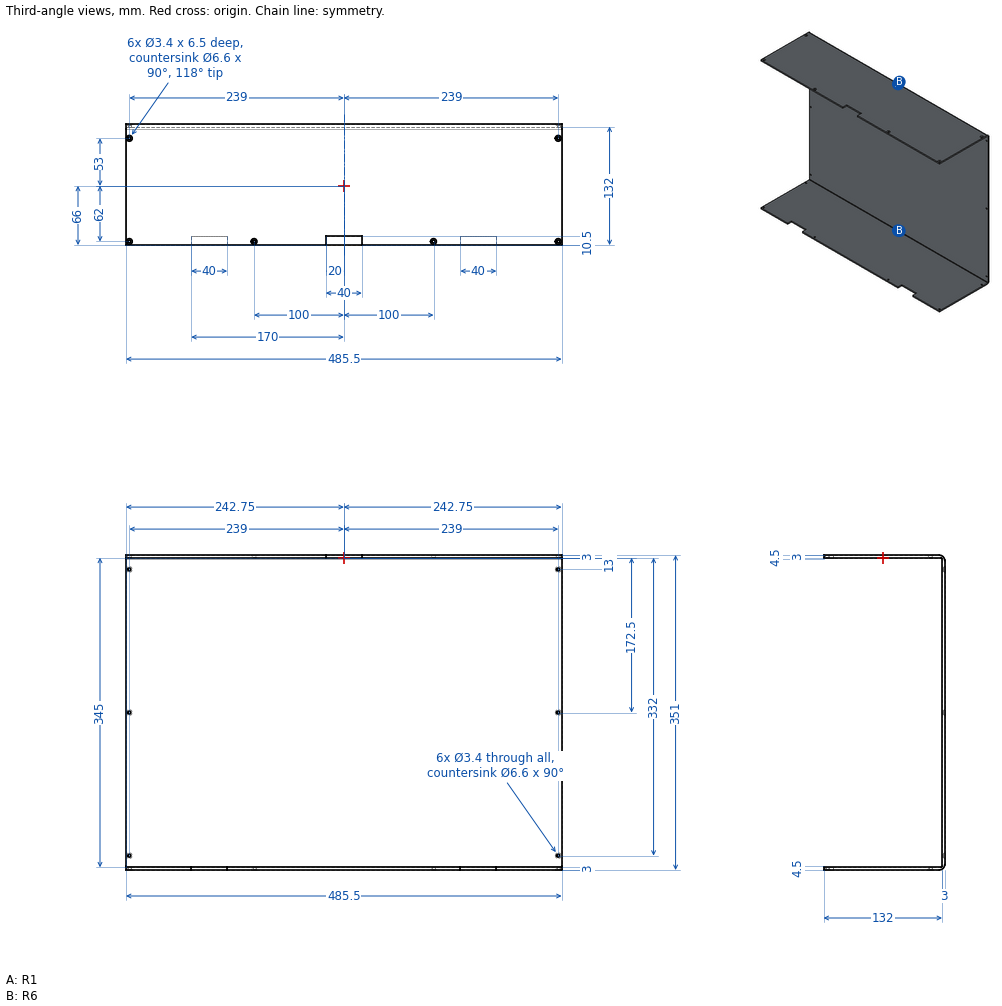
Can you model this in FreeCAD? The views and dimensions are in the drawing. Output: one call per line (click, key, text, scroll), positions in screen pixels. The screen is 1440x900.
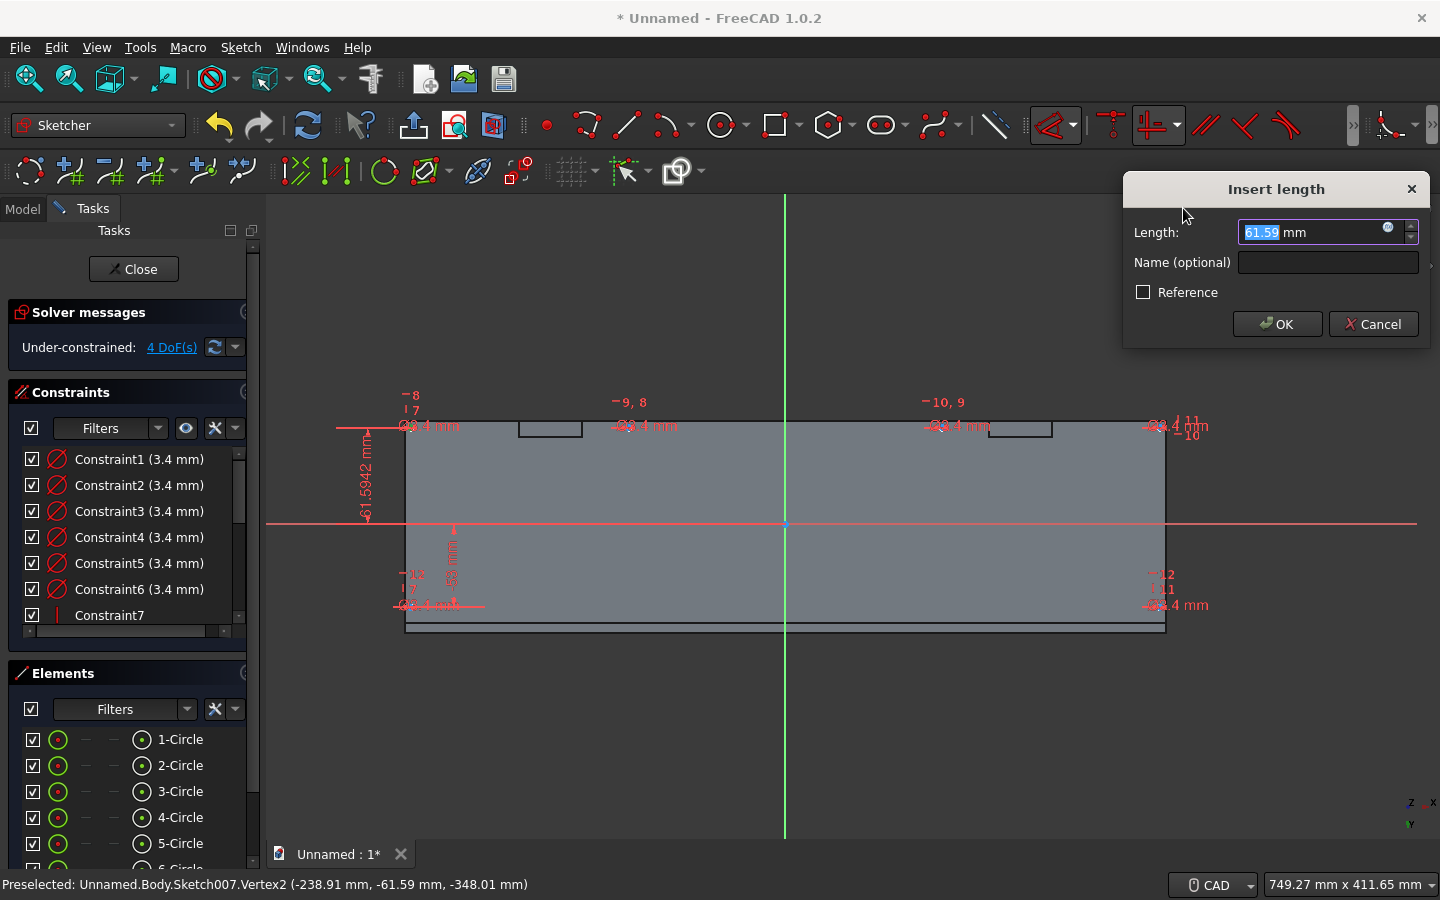
text(62)
key(Return)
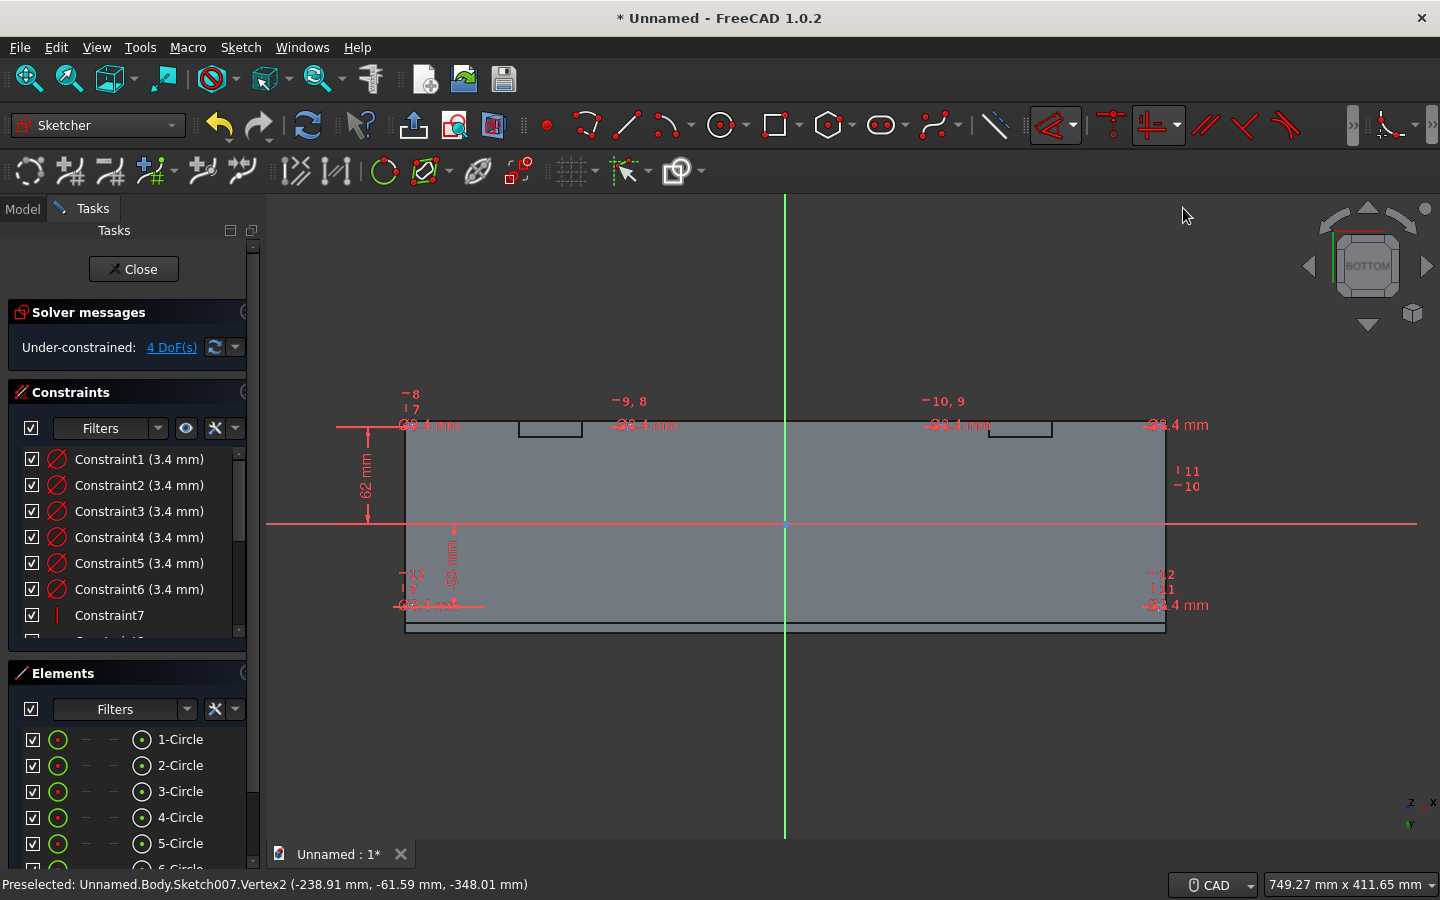
click(411, 607)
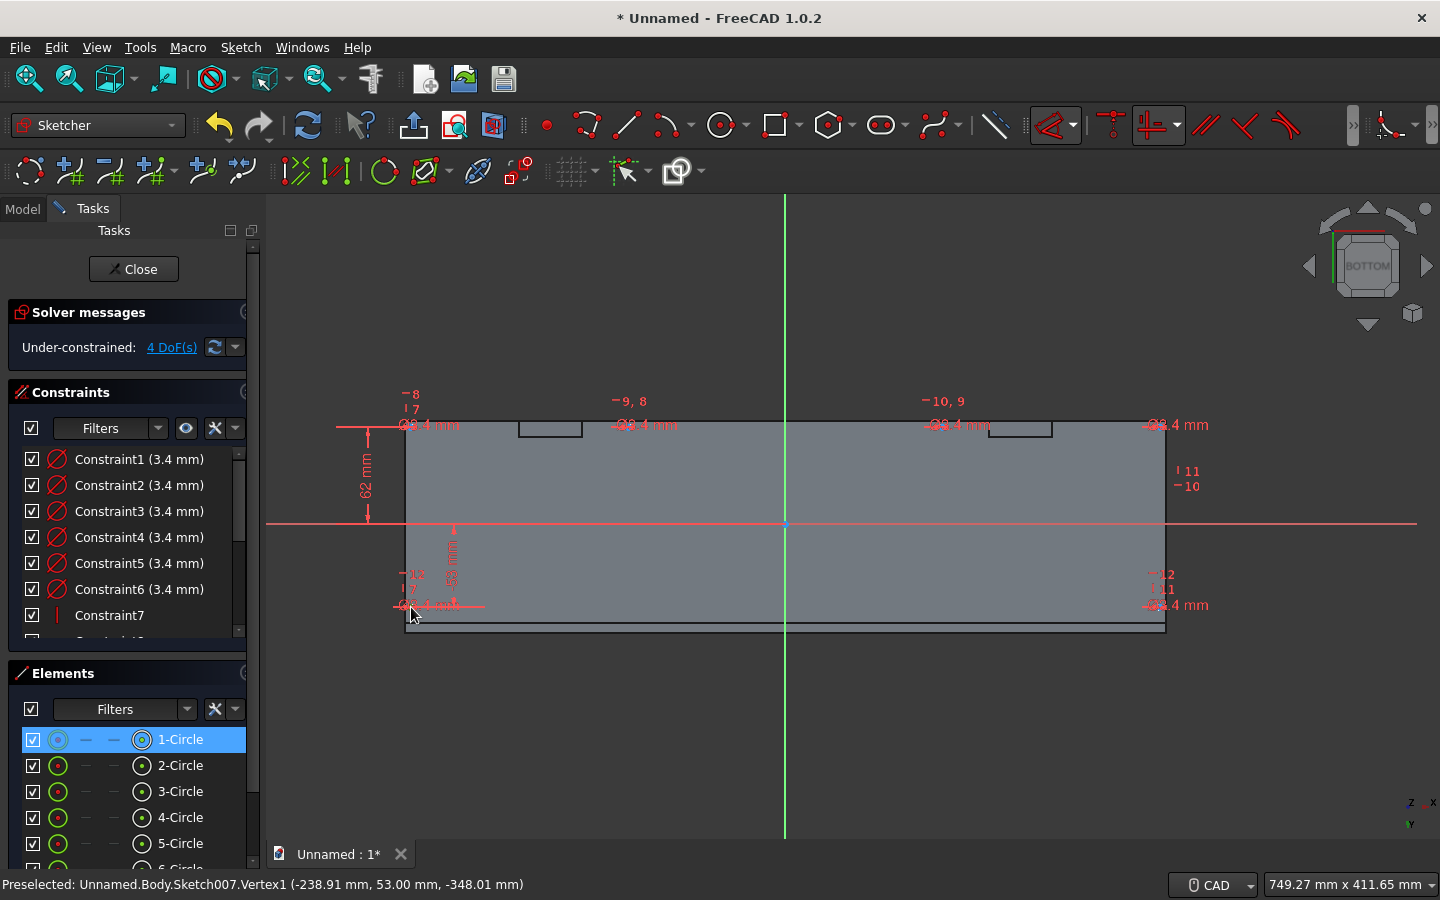
key(l)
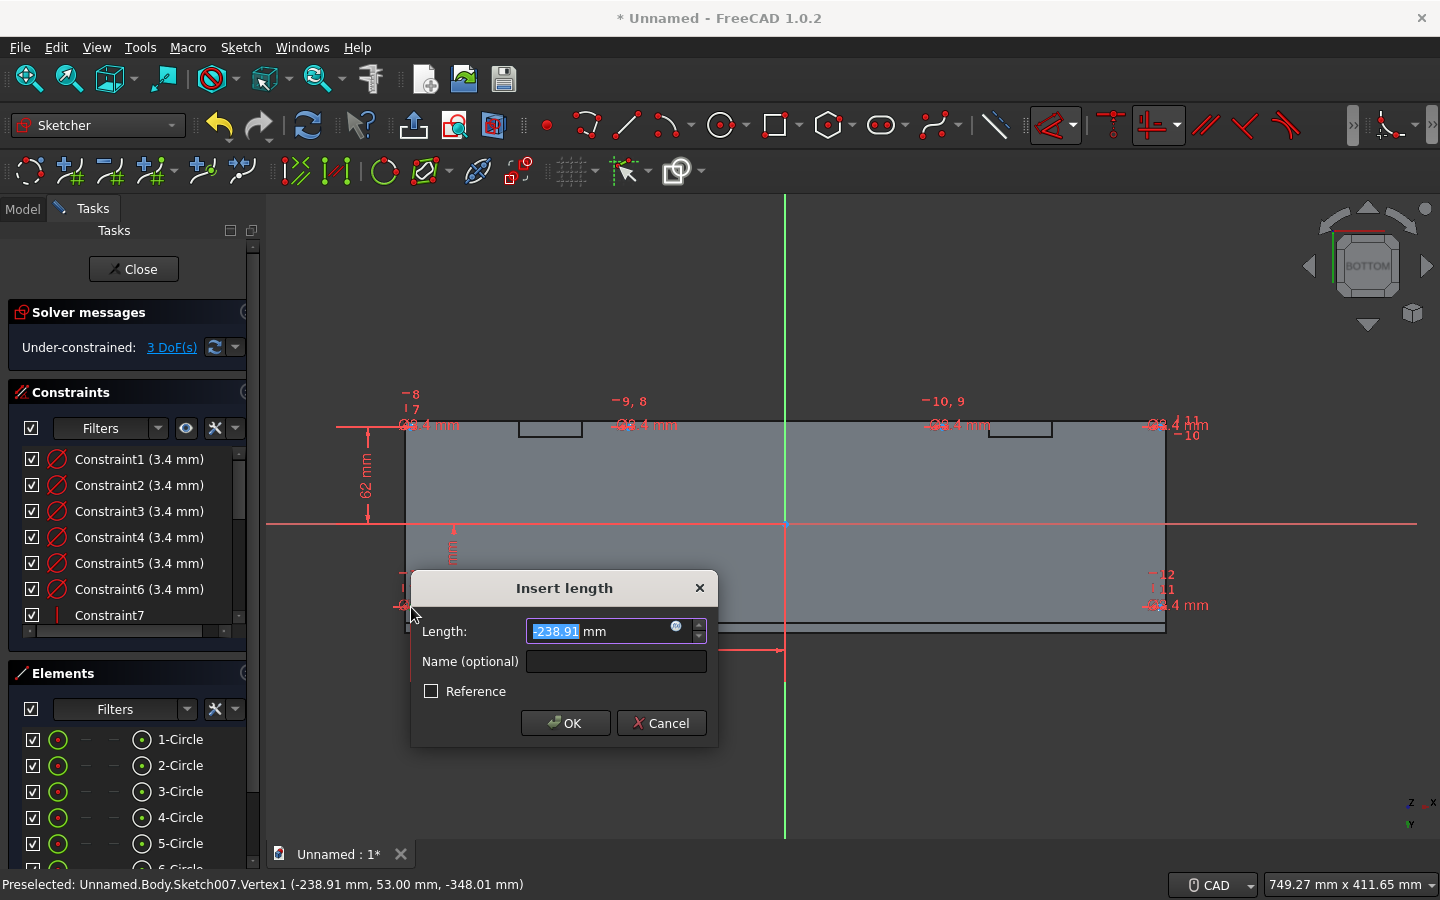
text(-239)
key(Return)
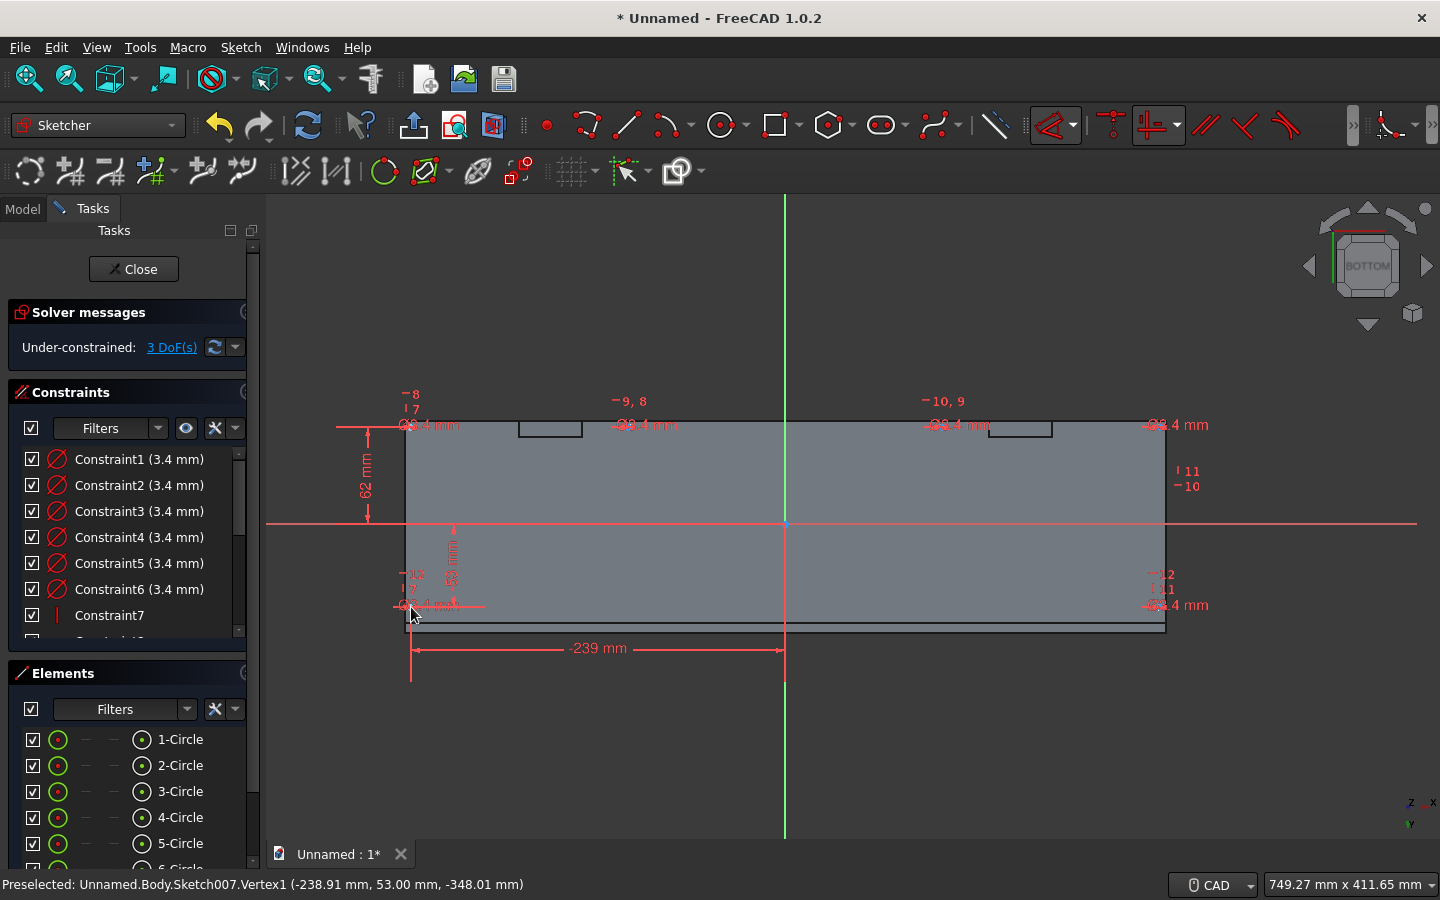
click(629, 427)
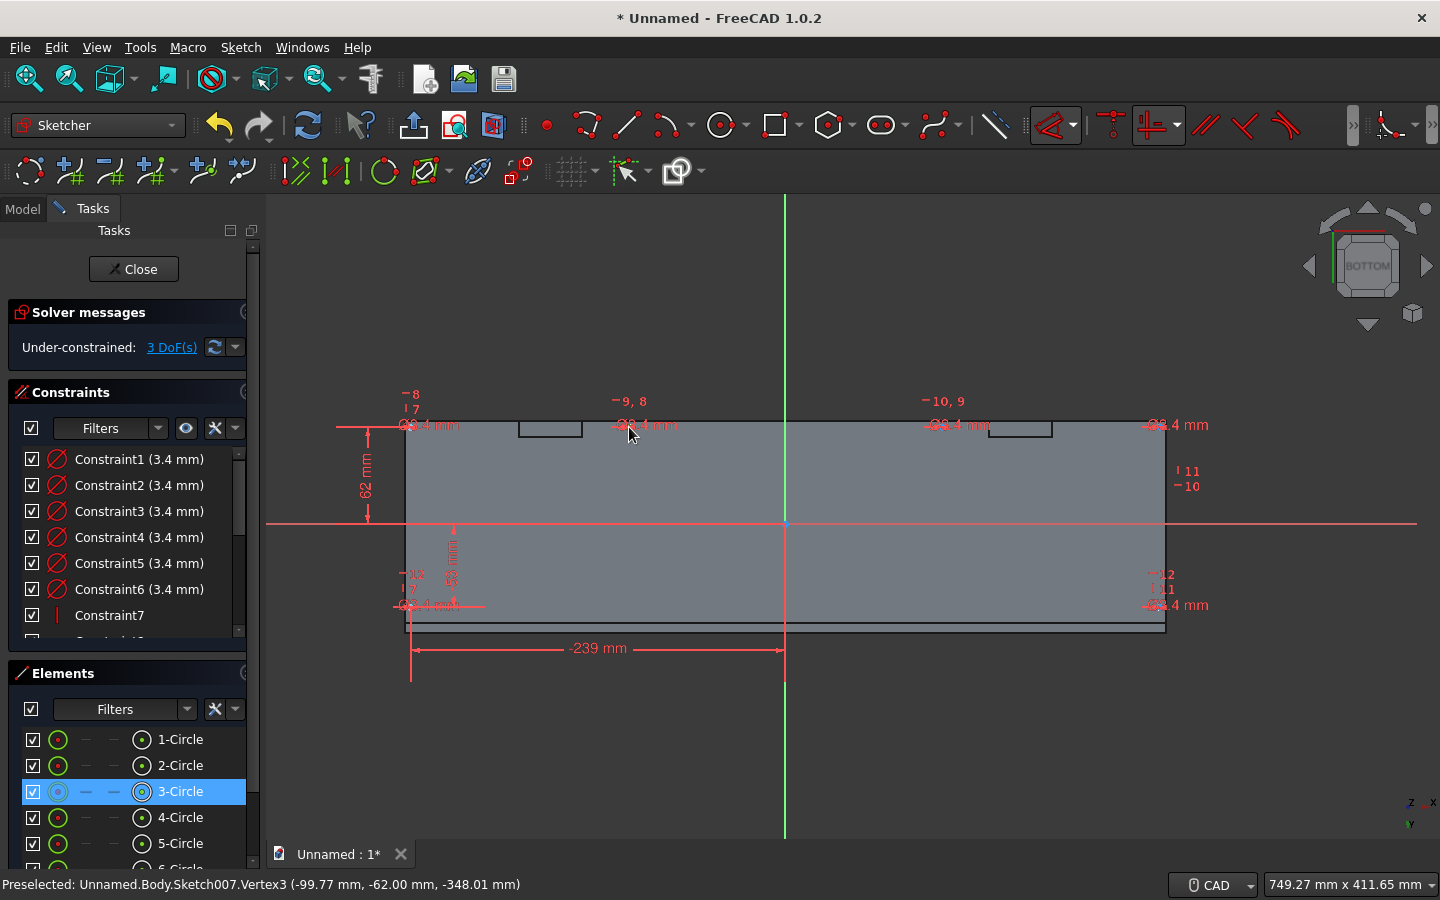
click(1076, 126)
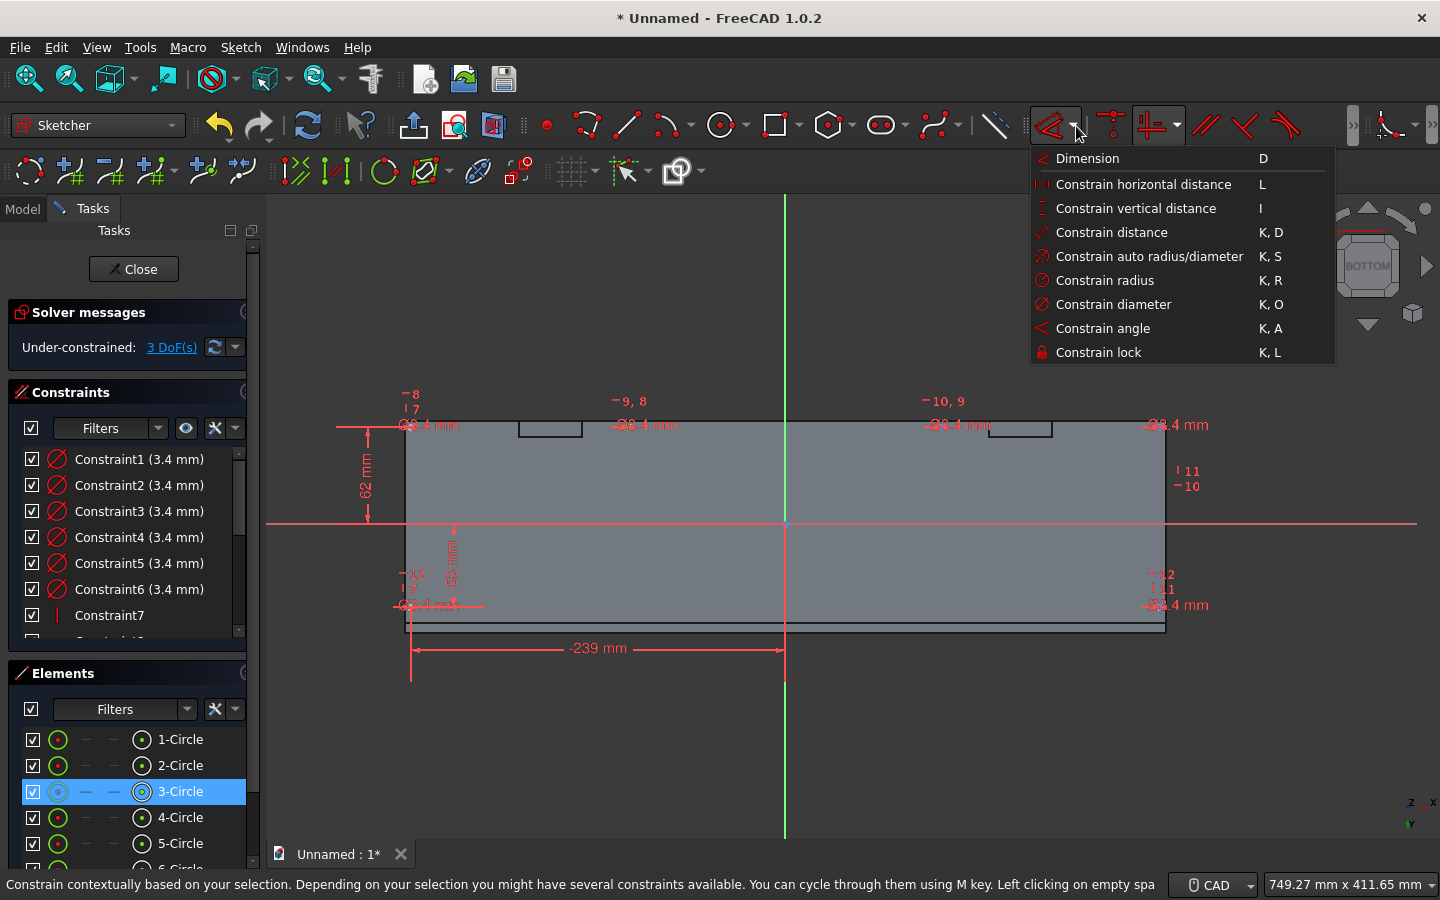
click(1183, 184)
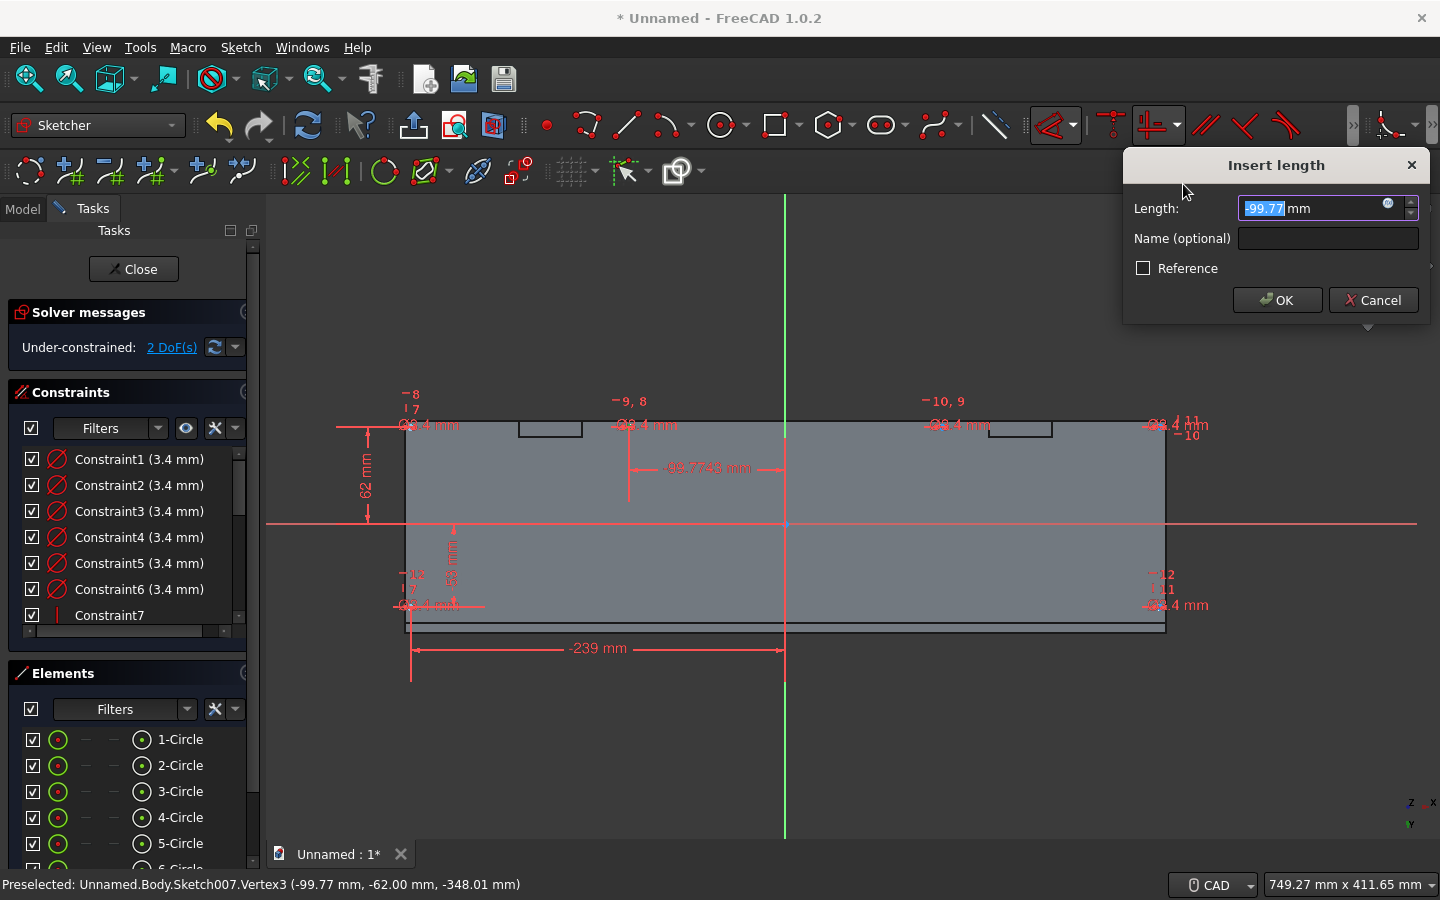
text(-100)
key(Return)